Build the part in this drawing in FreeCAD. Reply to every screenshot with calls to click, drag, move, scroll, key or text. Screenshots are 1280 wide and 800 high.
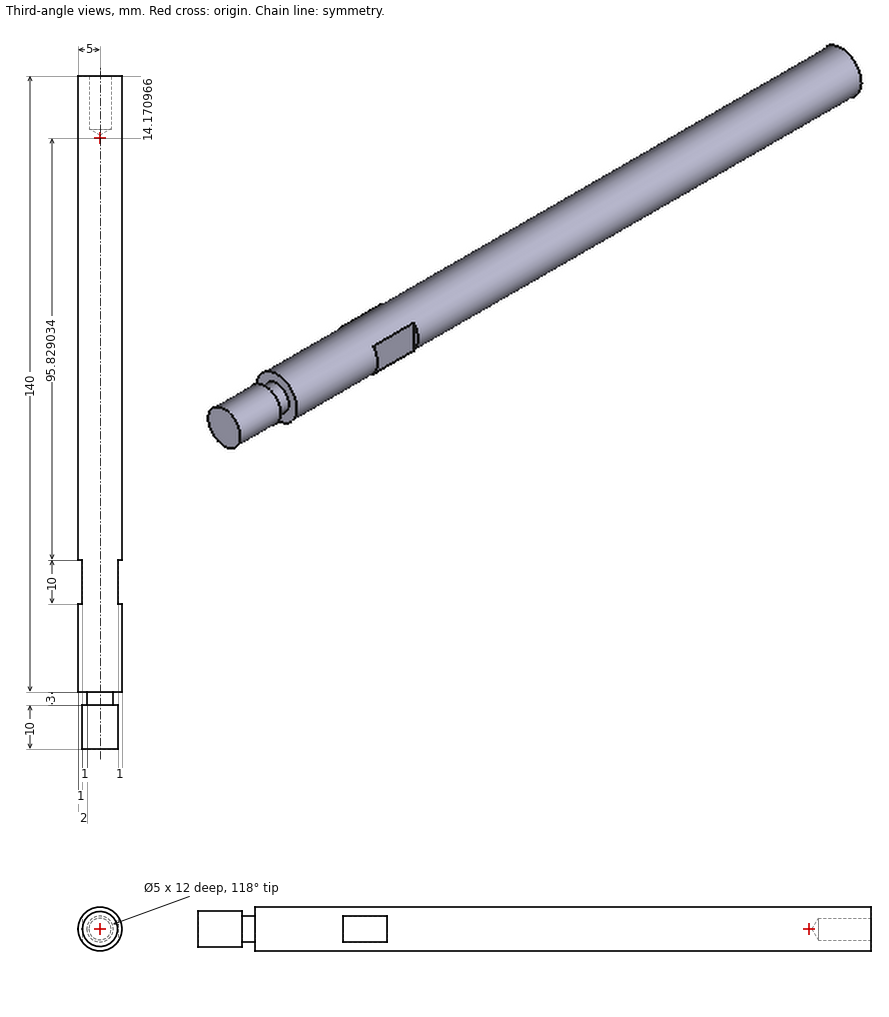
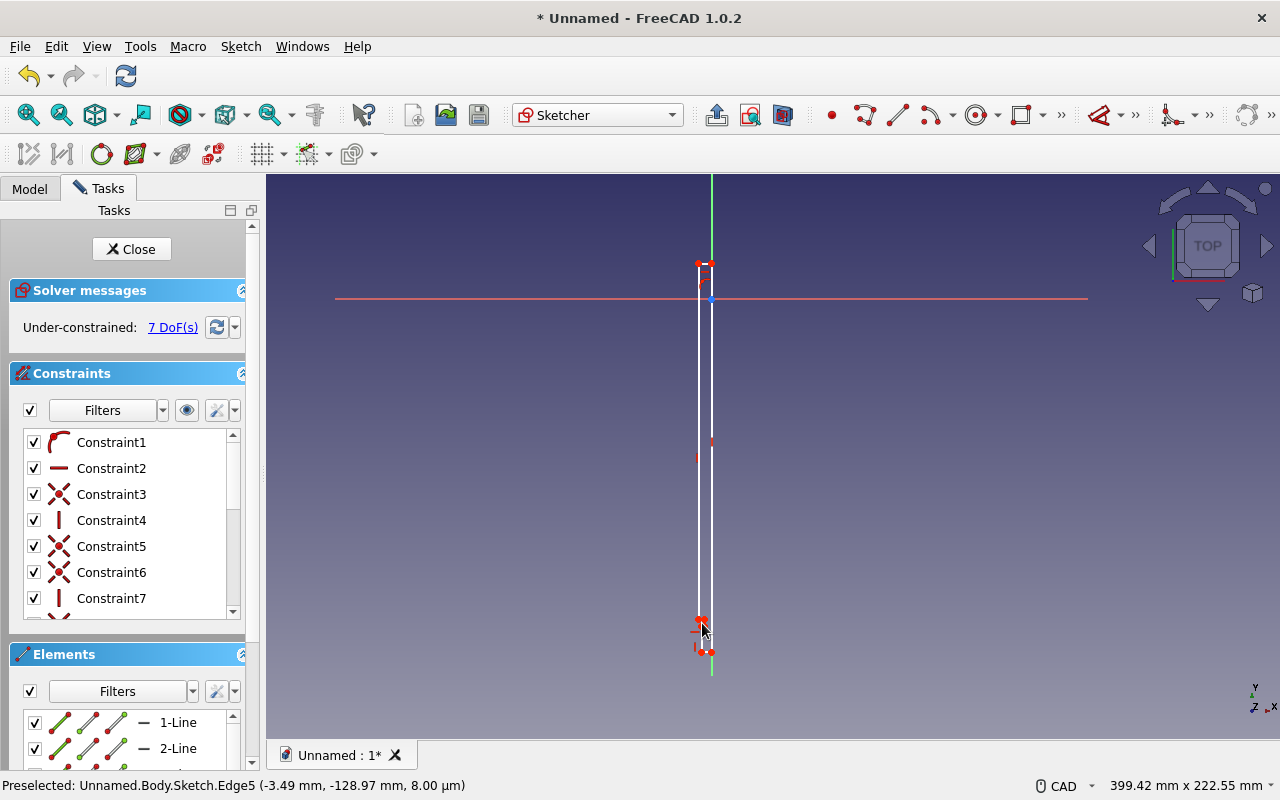
scroll(708, 264, up, 7)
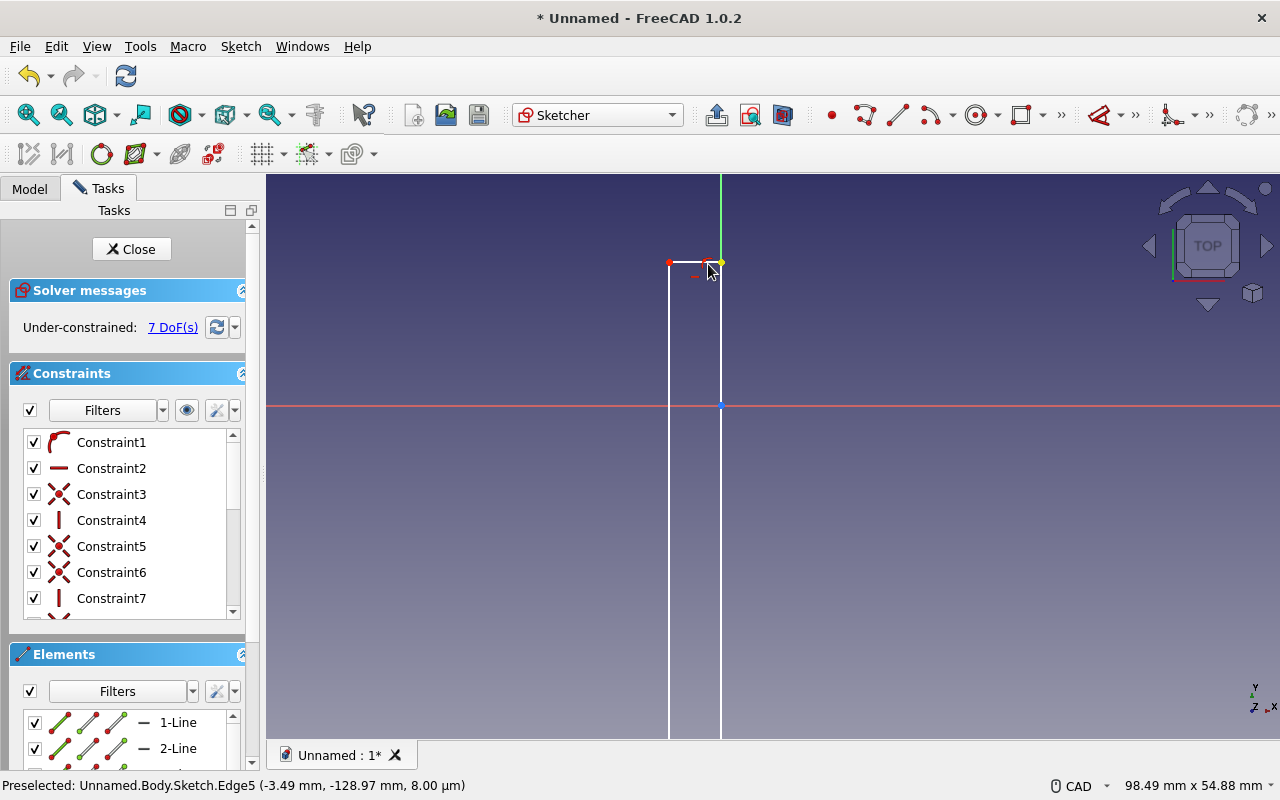
click(685, 262)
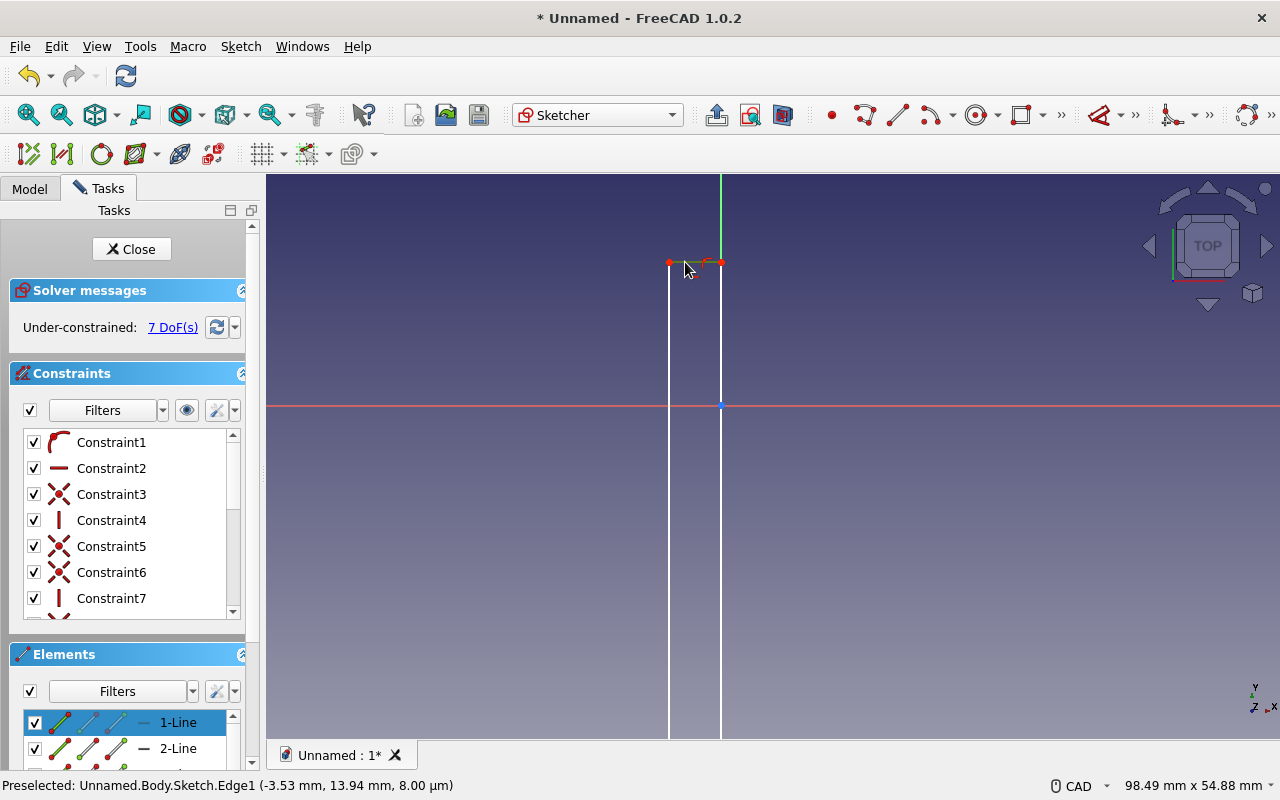
click(1120, 116)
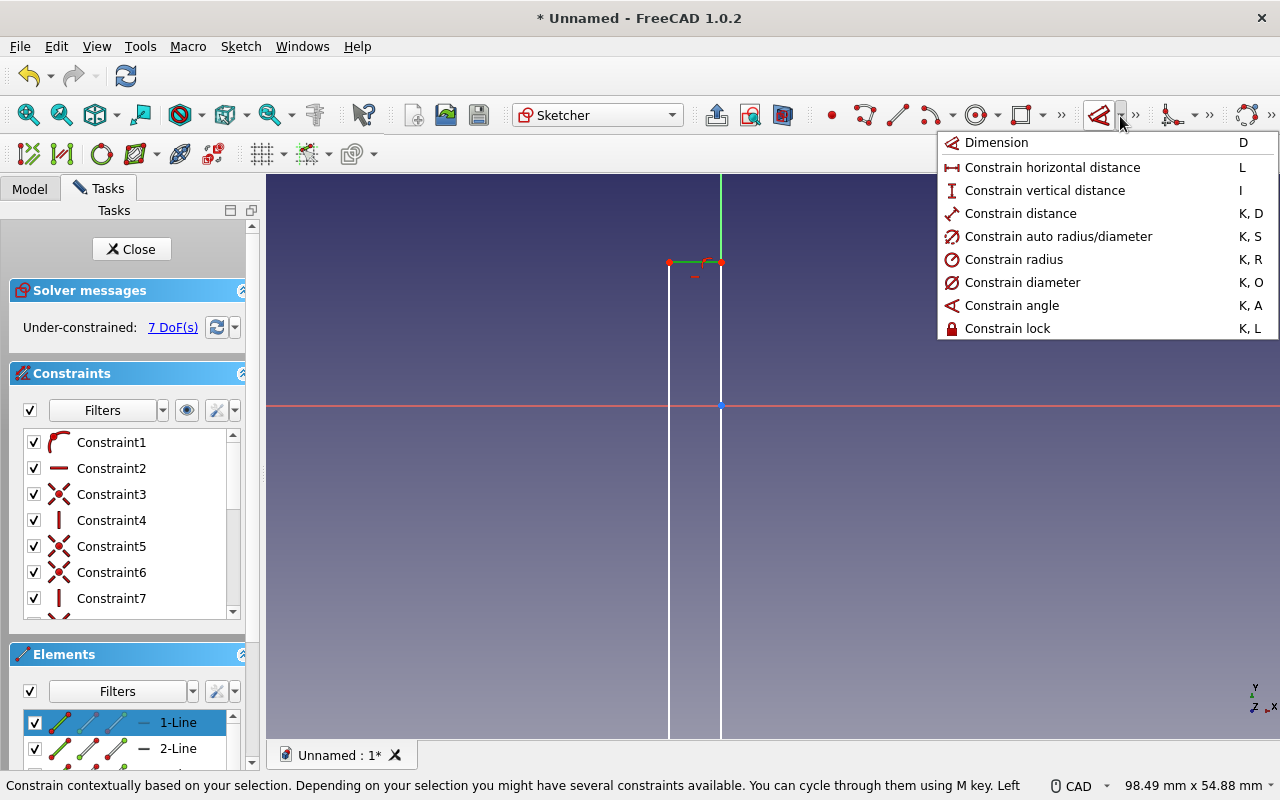
click(1108, 168)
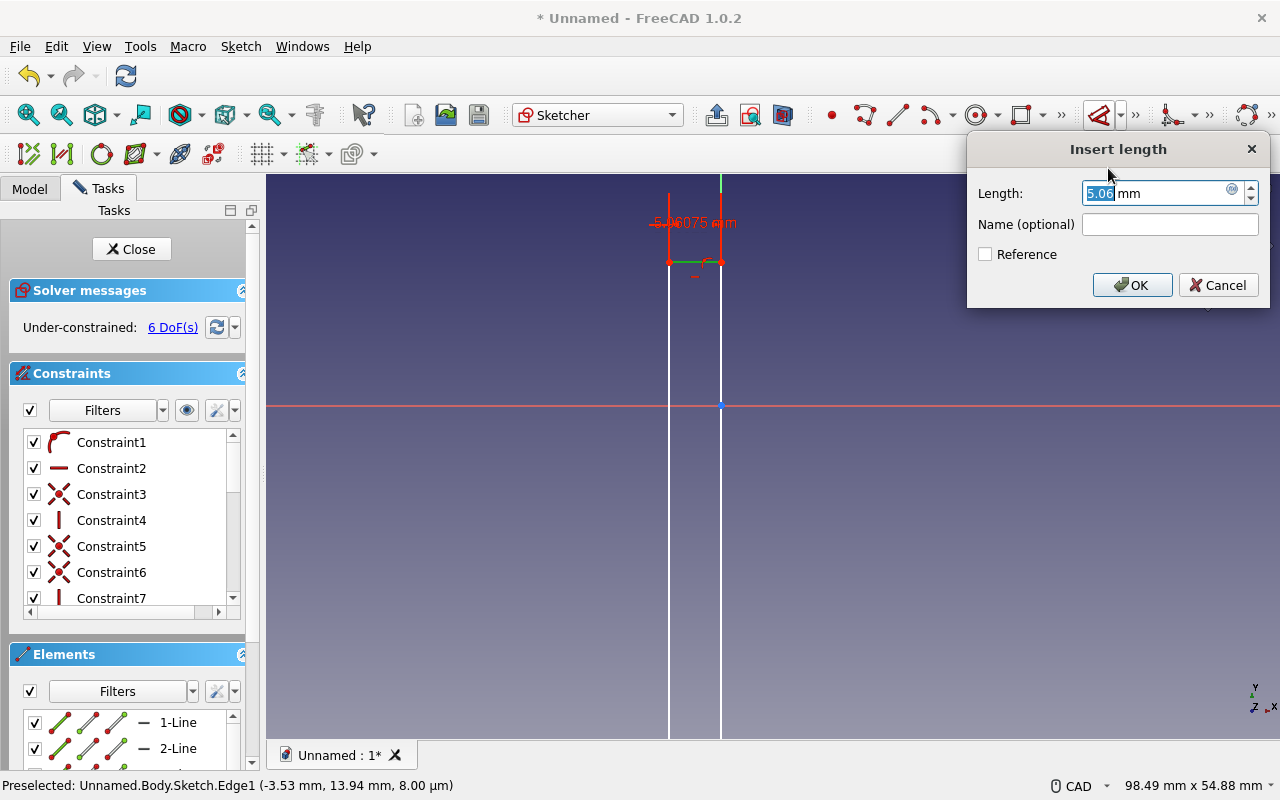
text(5)
key(Return)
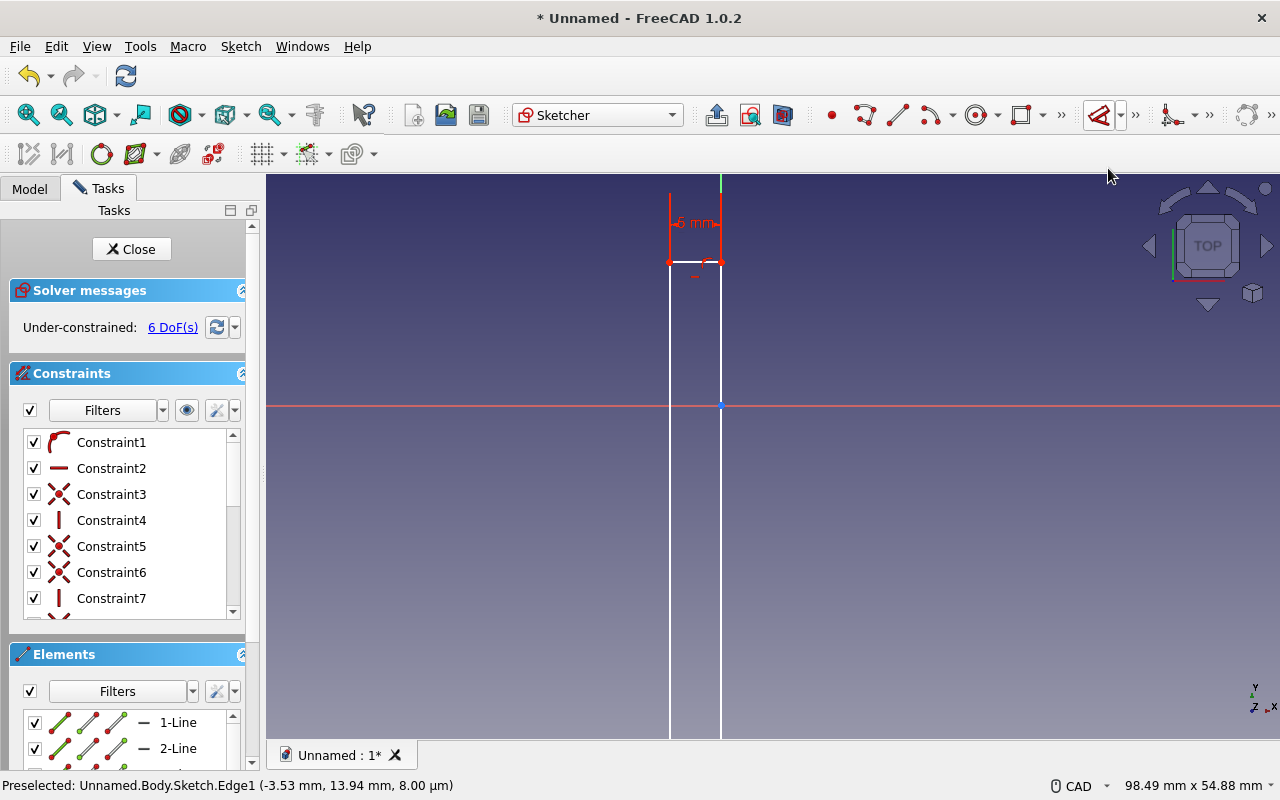
scroll(707, 263, down, 7)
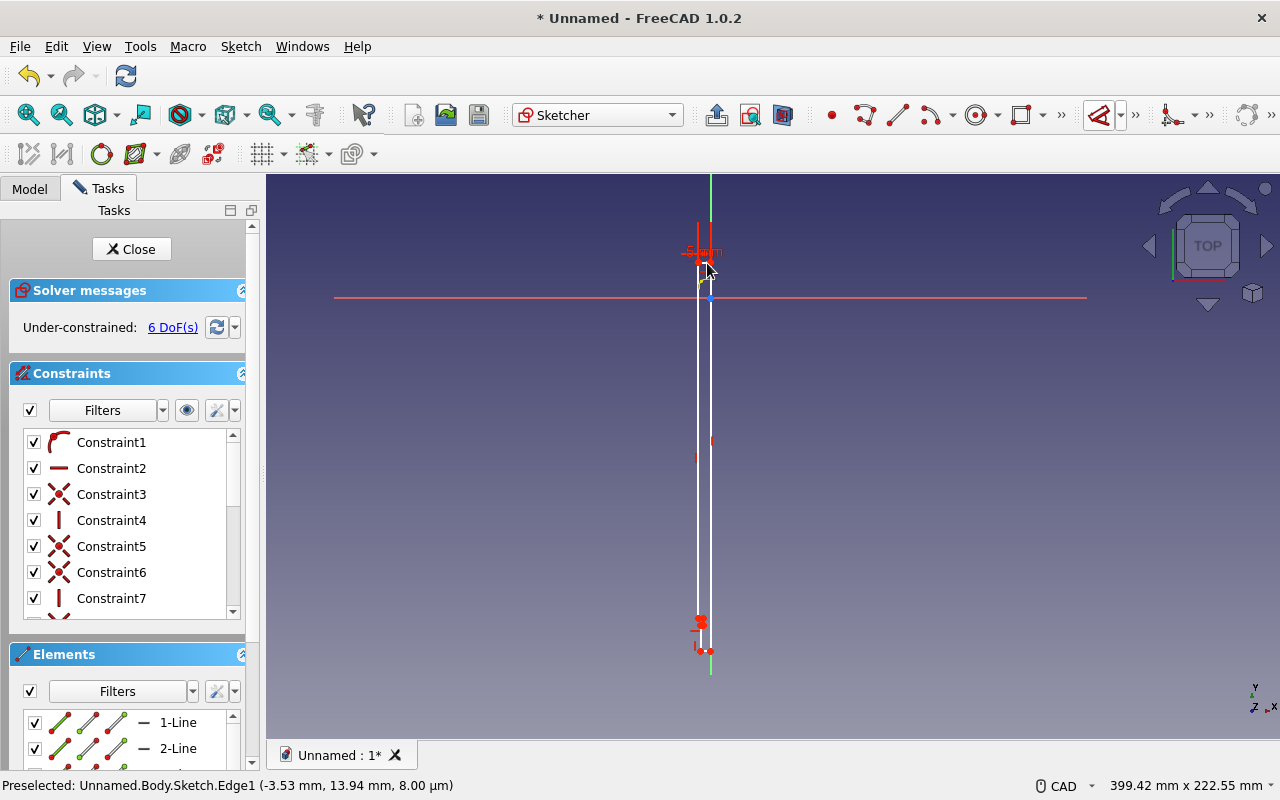
scroll(701, 618, up, 11)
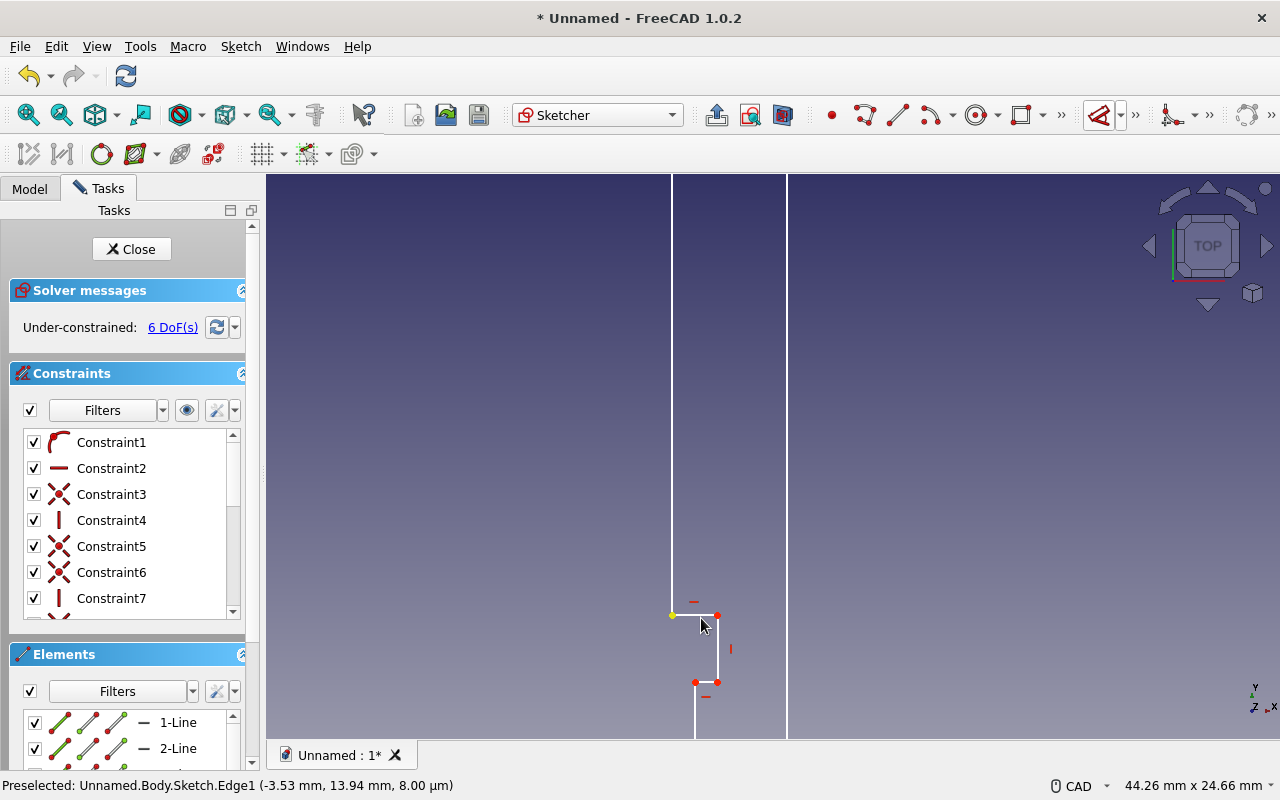
click(695, 615)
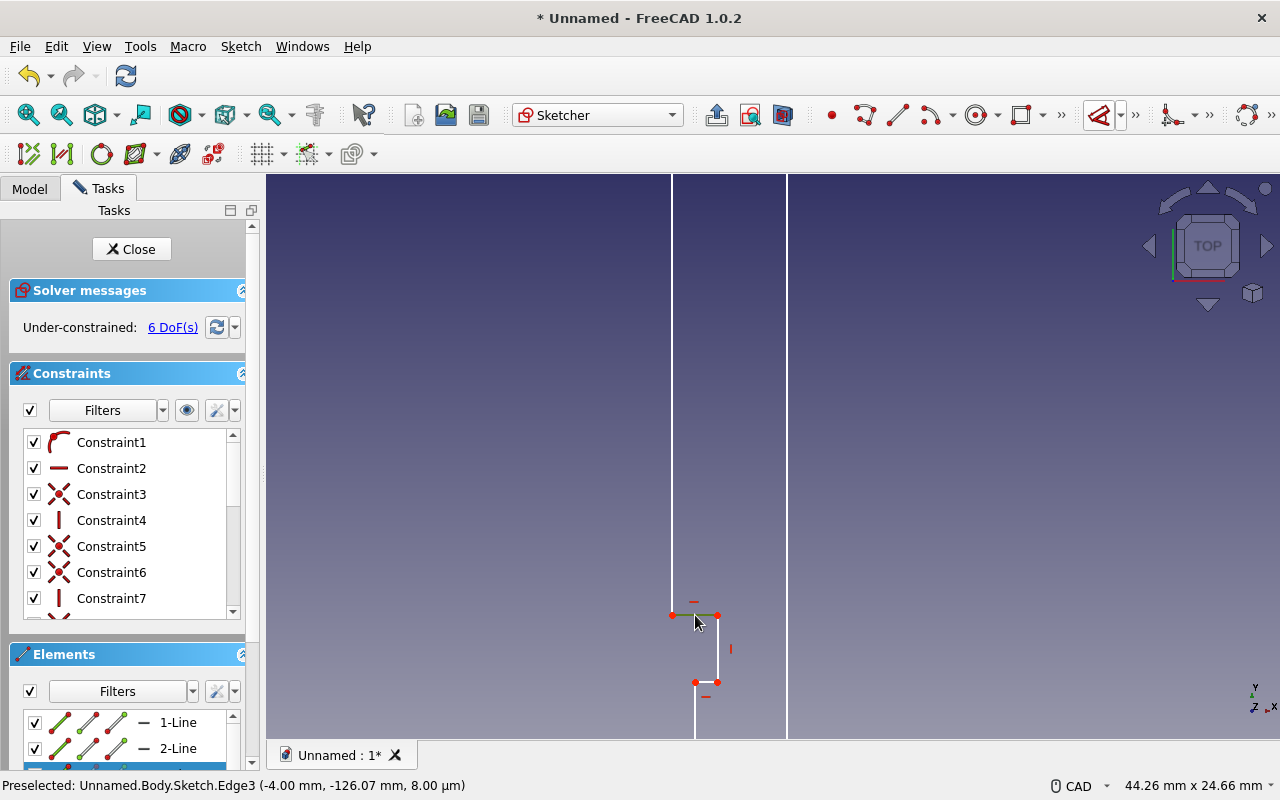
key(l)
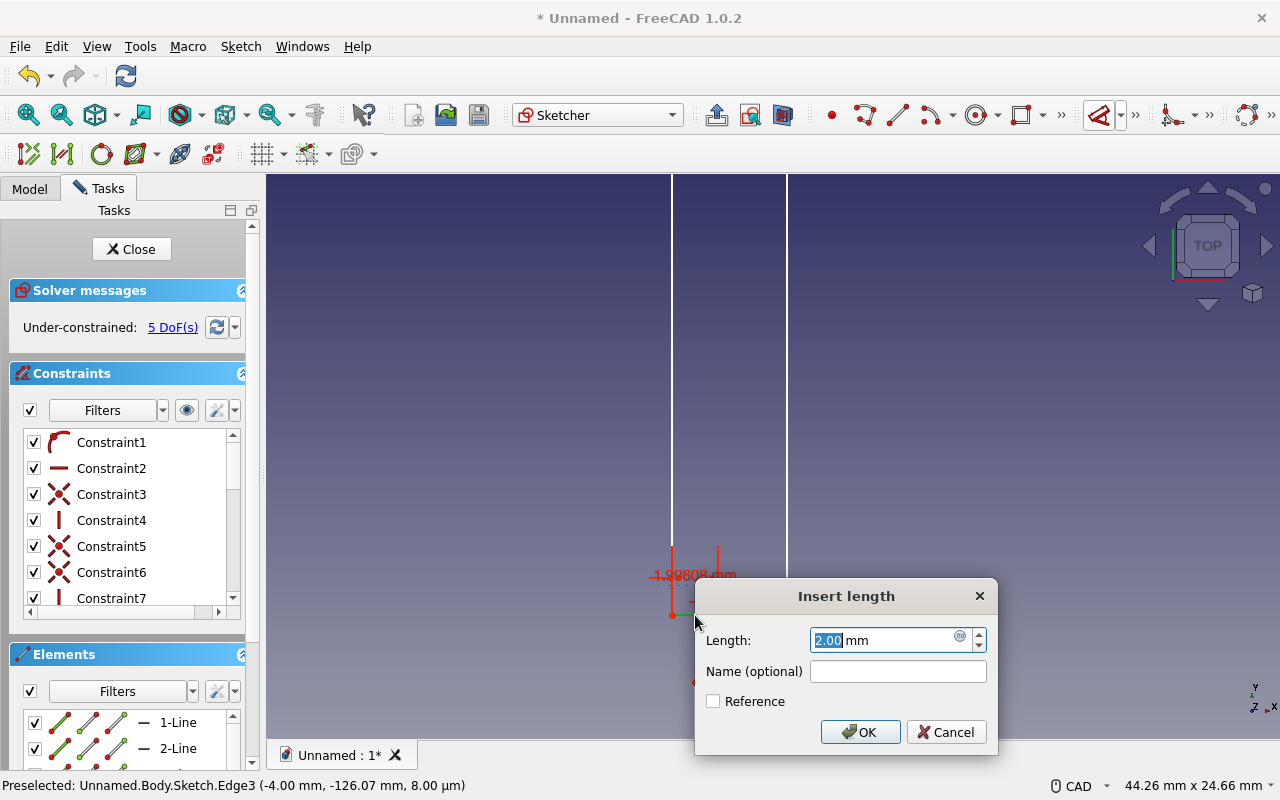
text(2)
key(Return)